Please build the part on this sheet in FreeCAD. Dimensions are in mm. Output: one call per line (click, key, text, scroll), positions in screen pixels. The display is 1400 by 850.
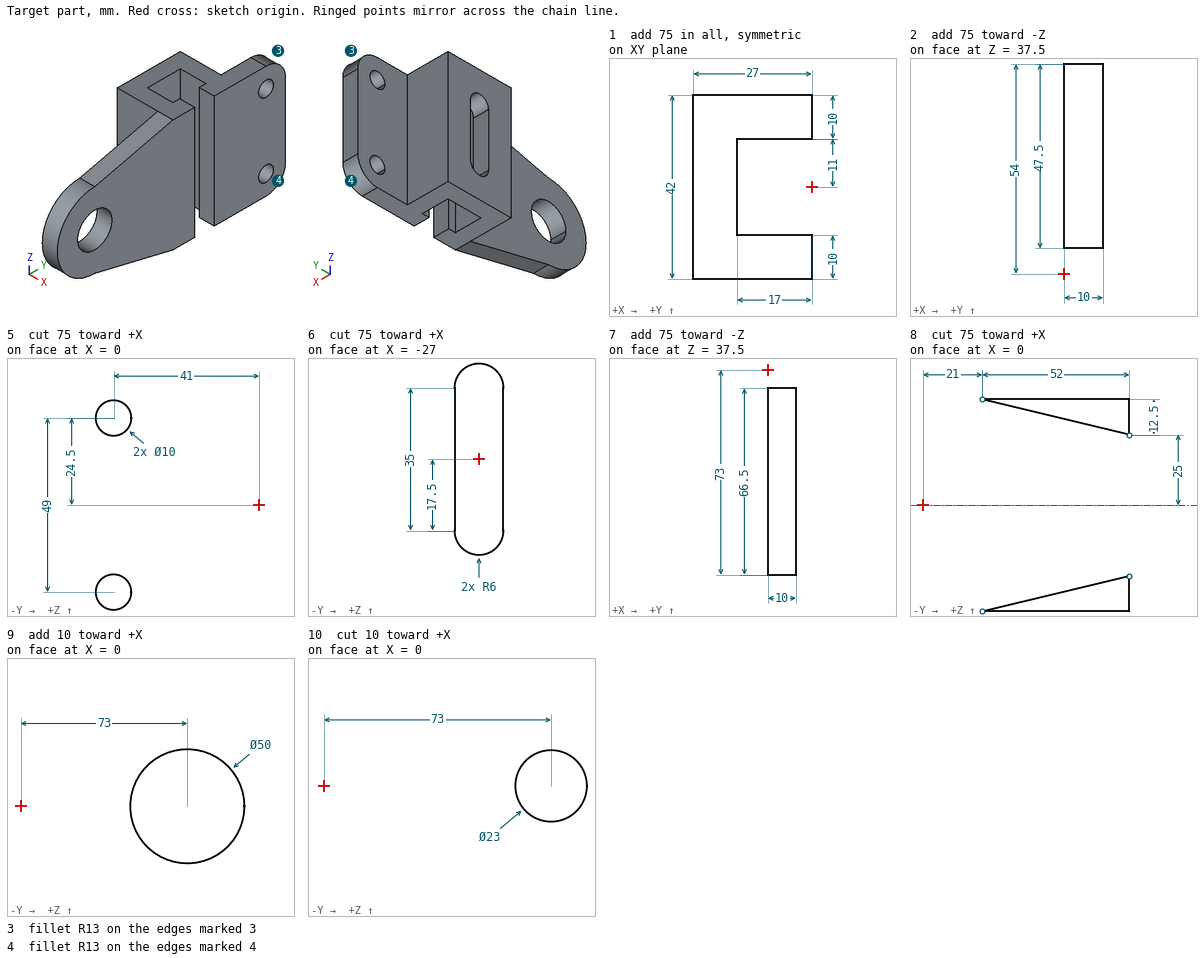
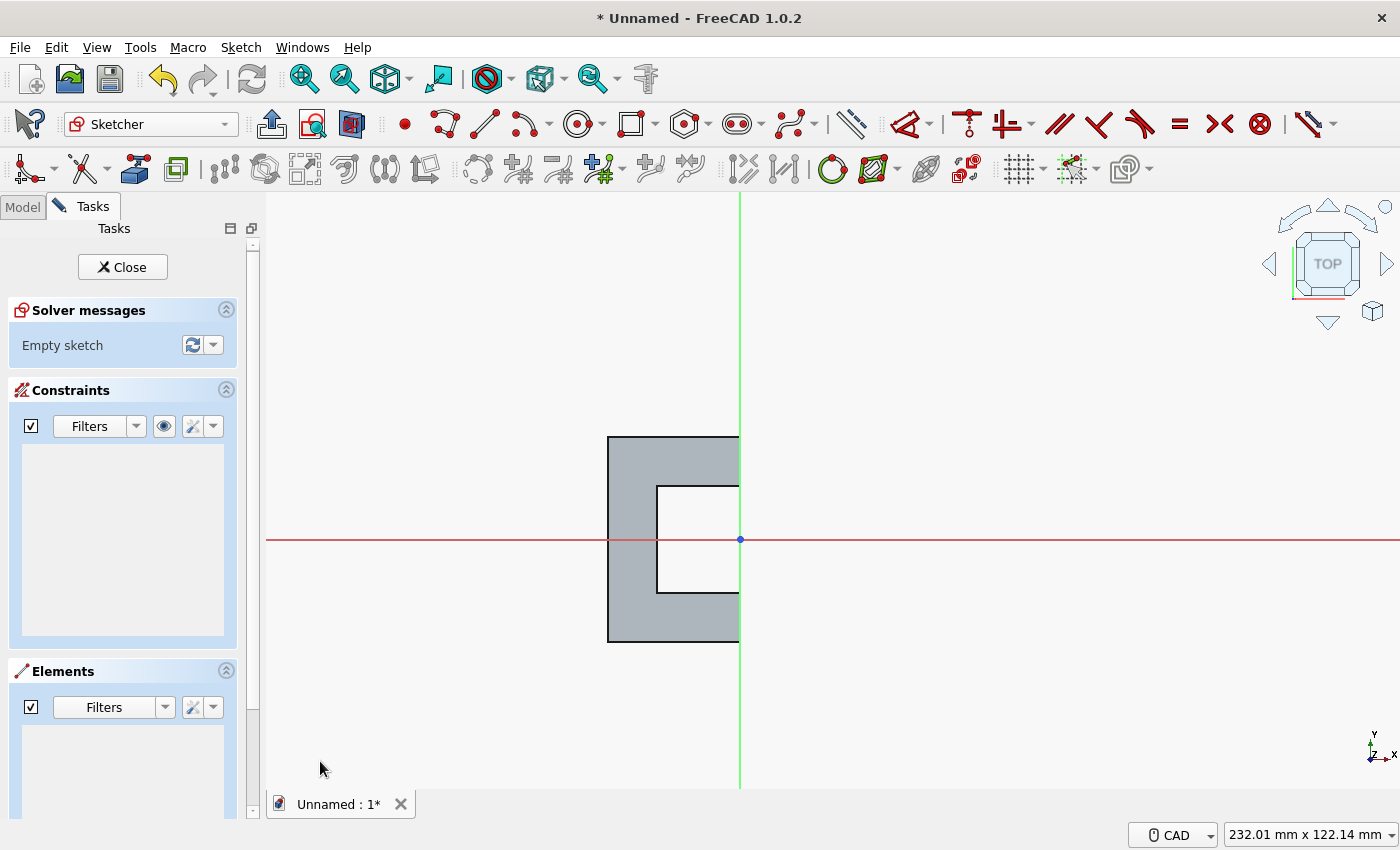
scroll(764, 239, up, 2)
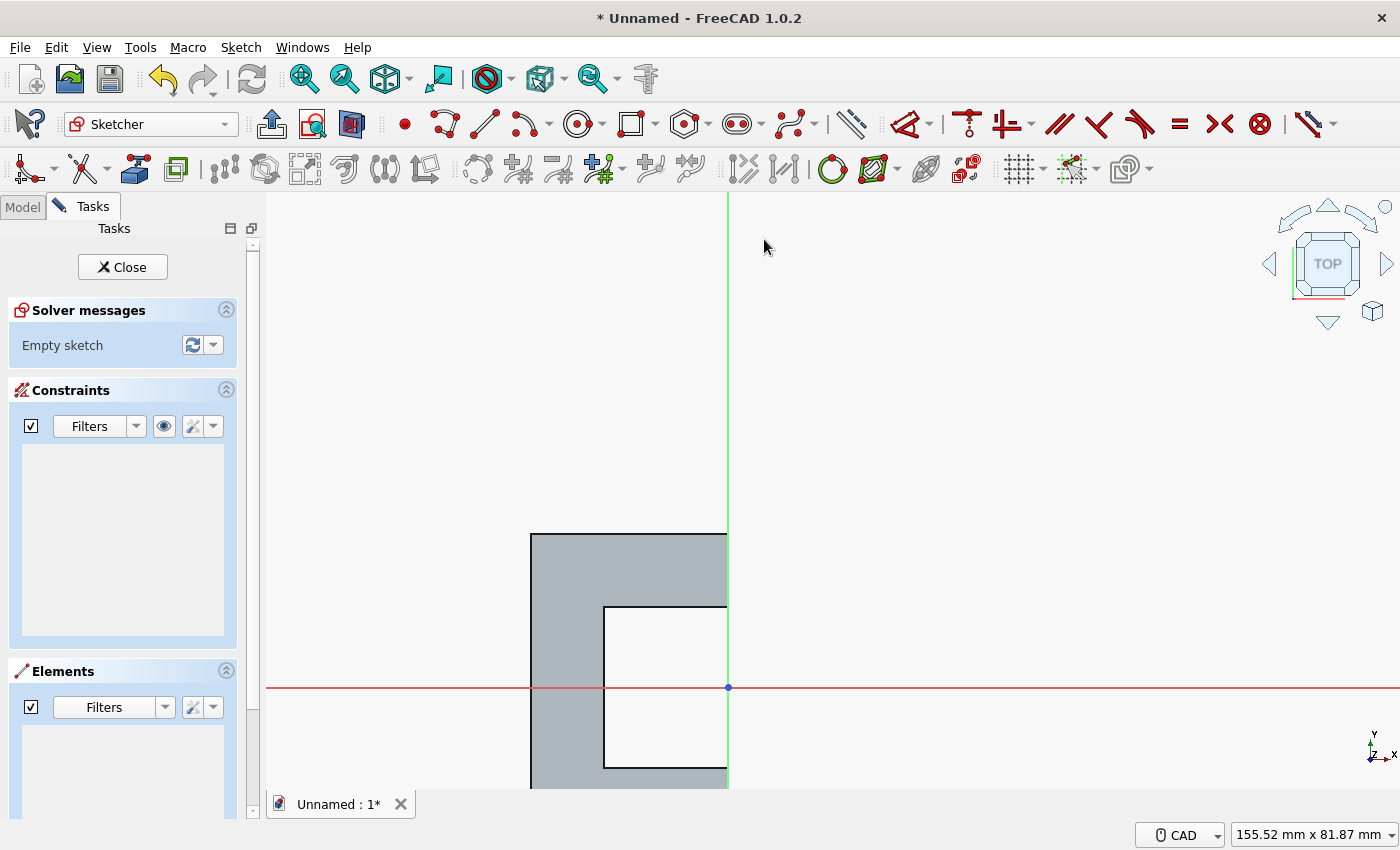
key(g)
key(r)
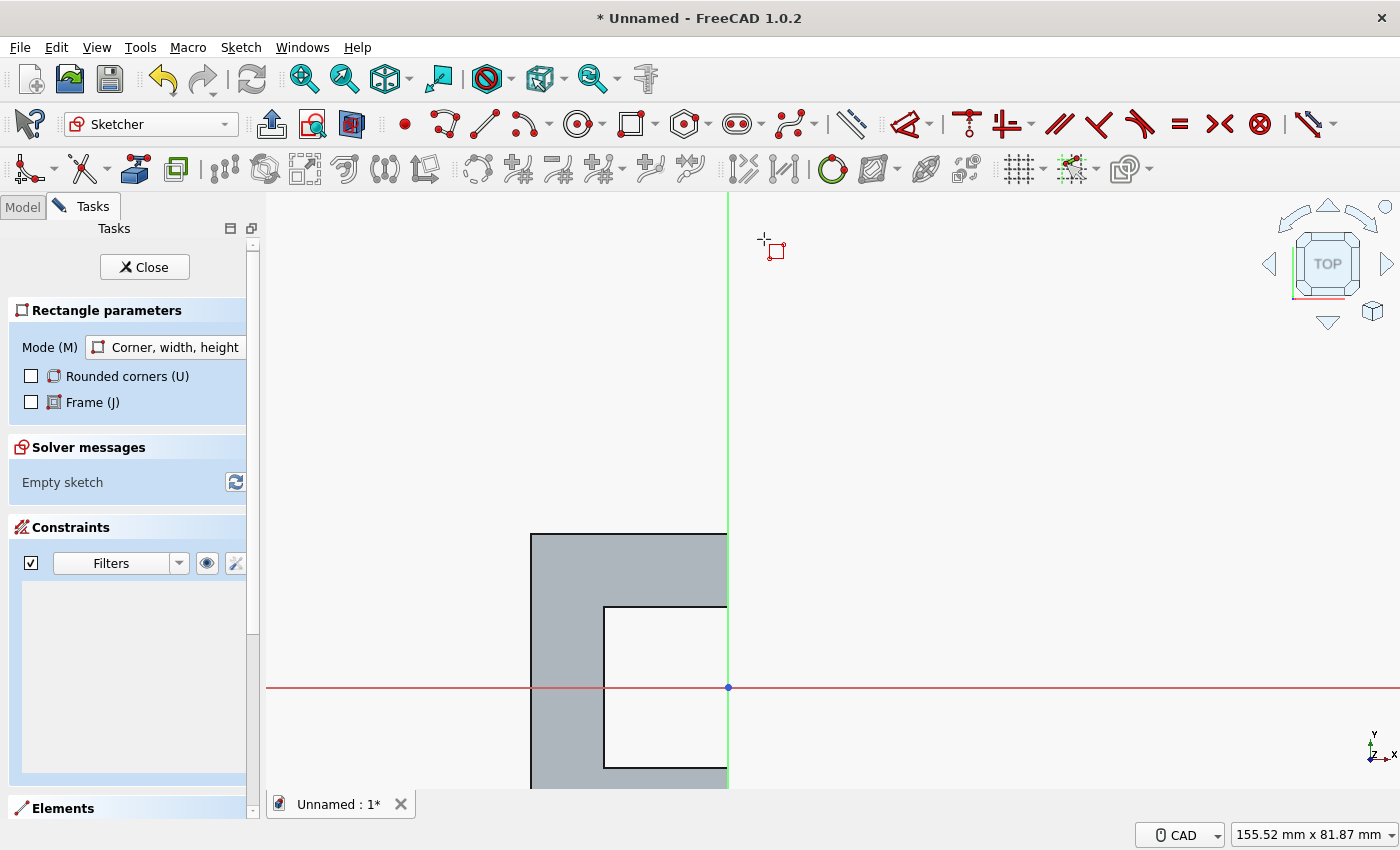
click(728, 294)
click(801, 640)
key(Escape)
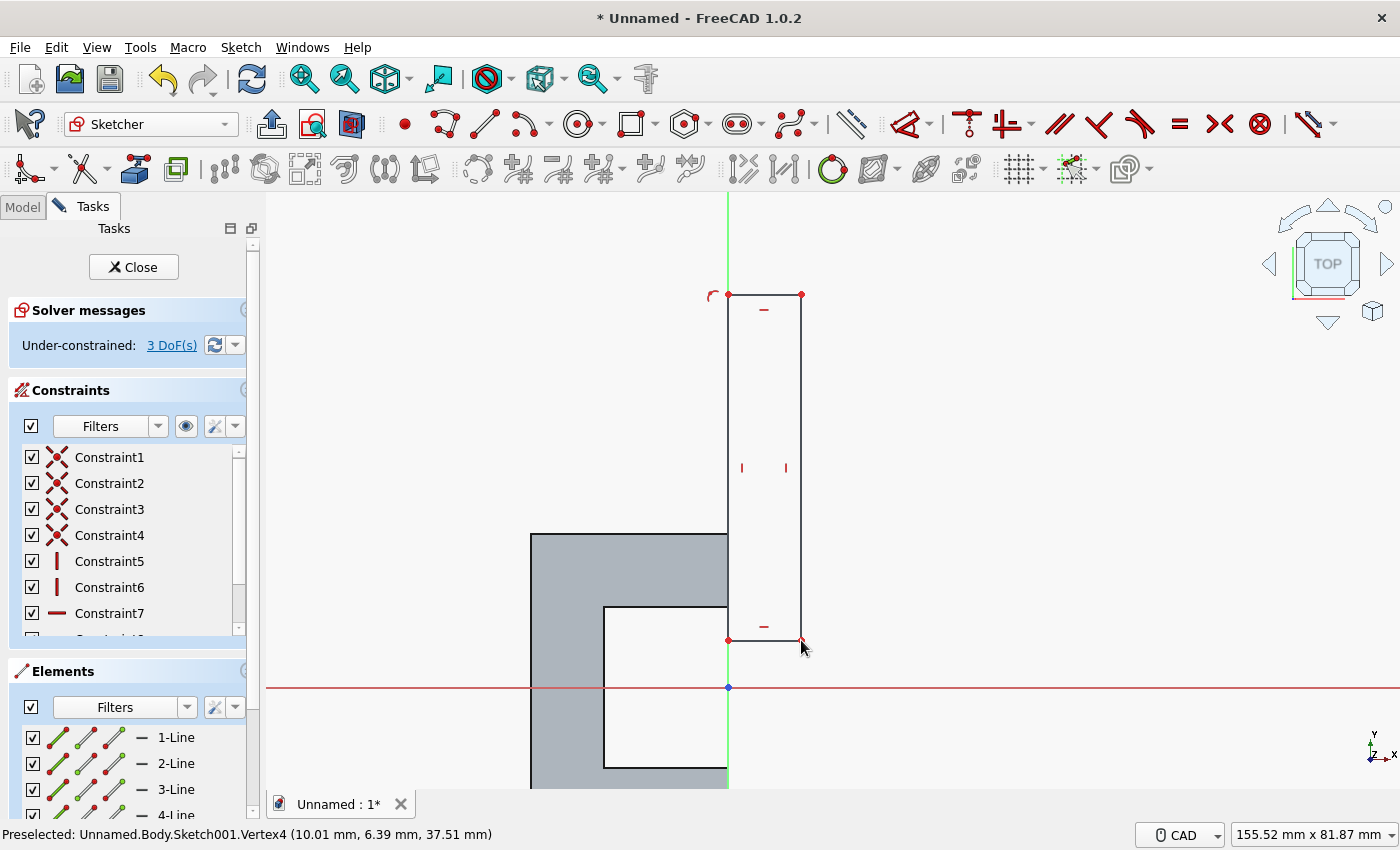
key(d)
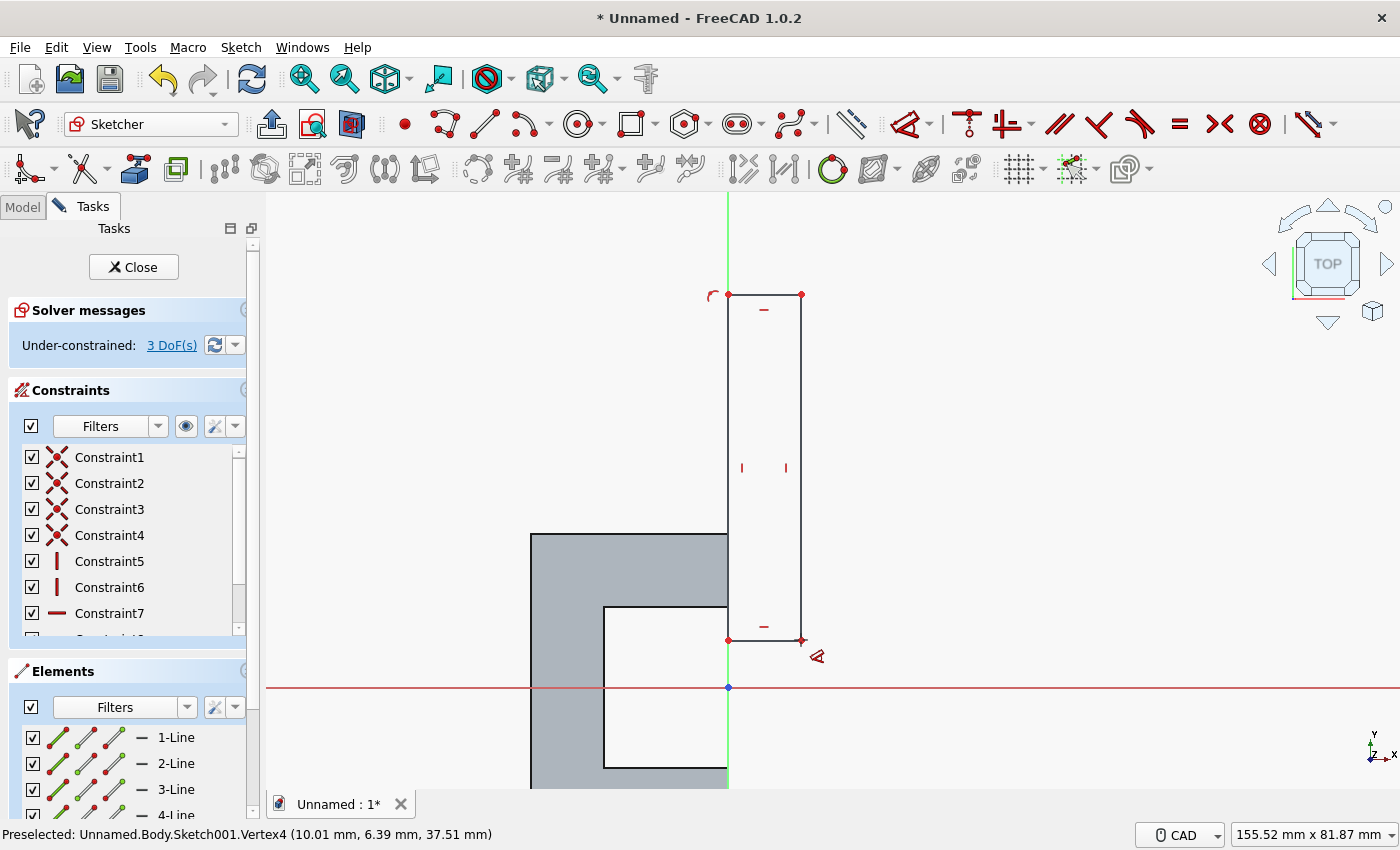
click(750, 641)
click(765, 607)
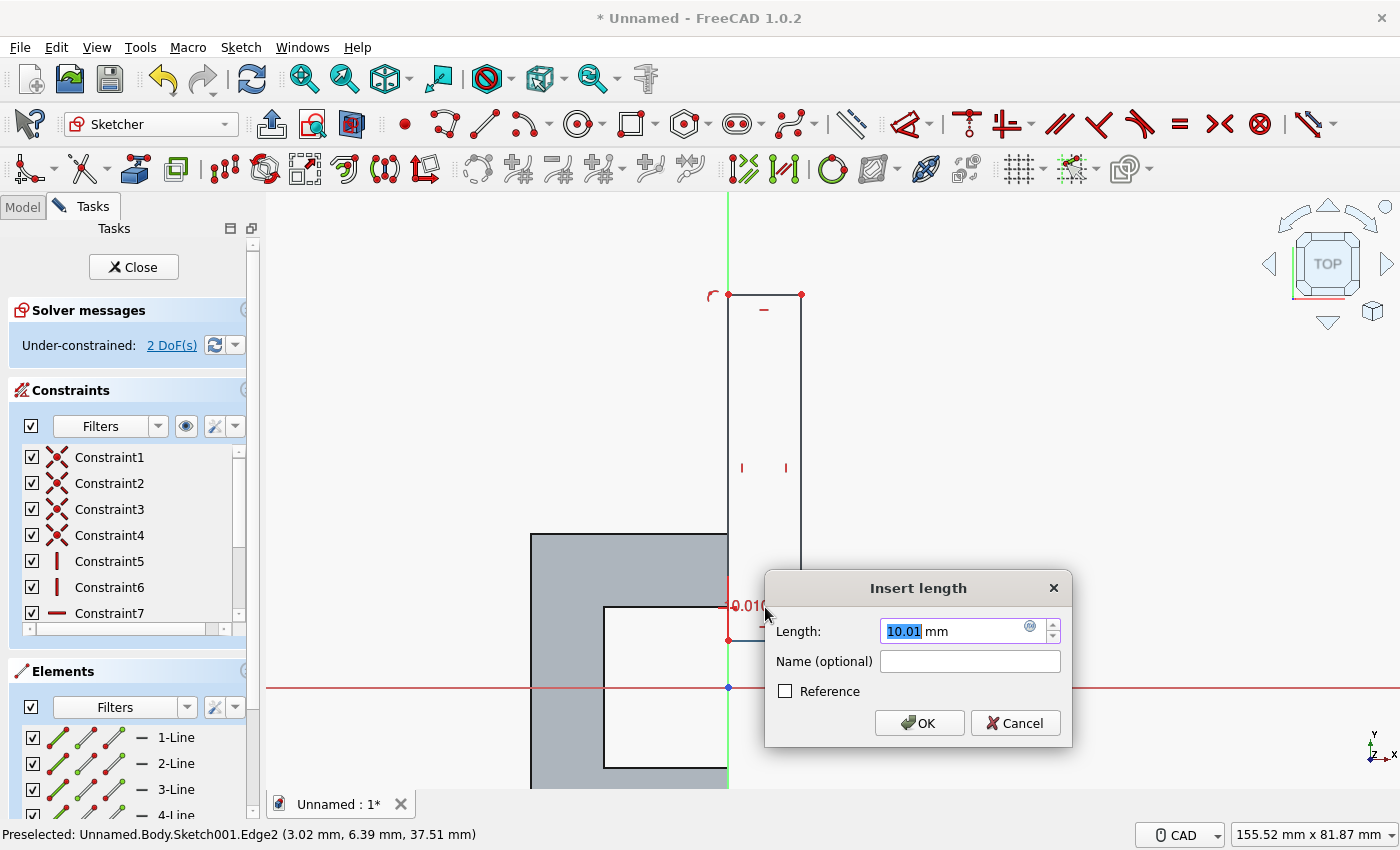
text(10)
key(Return)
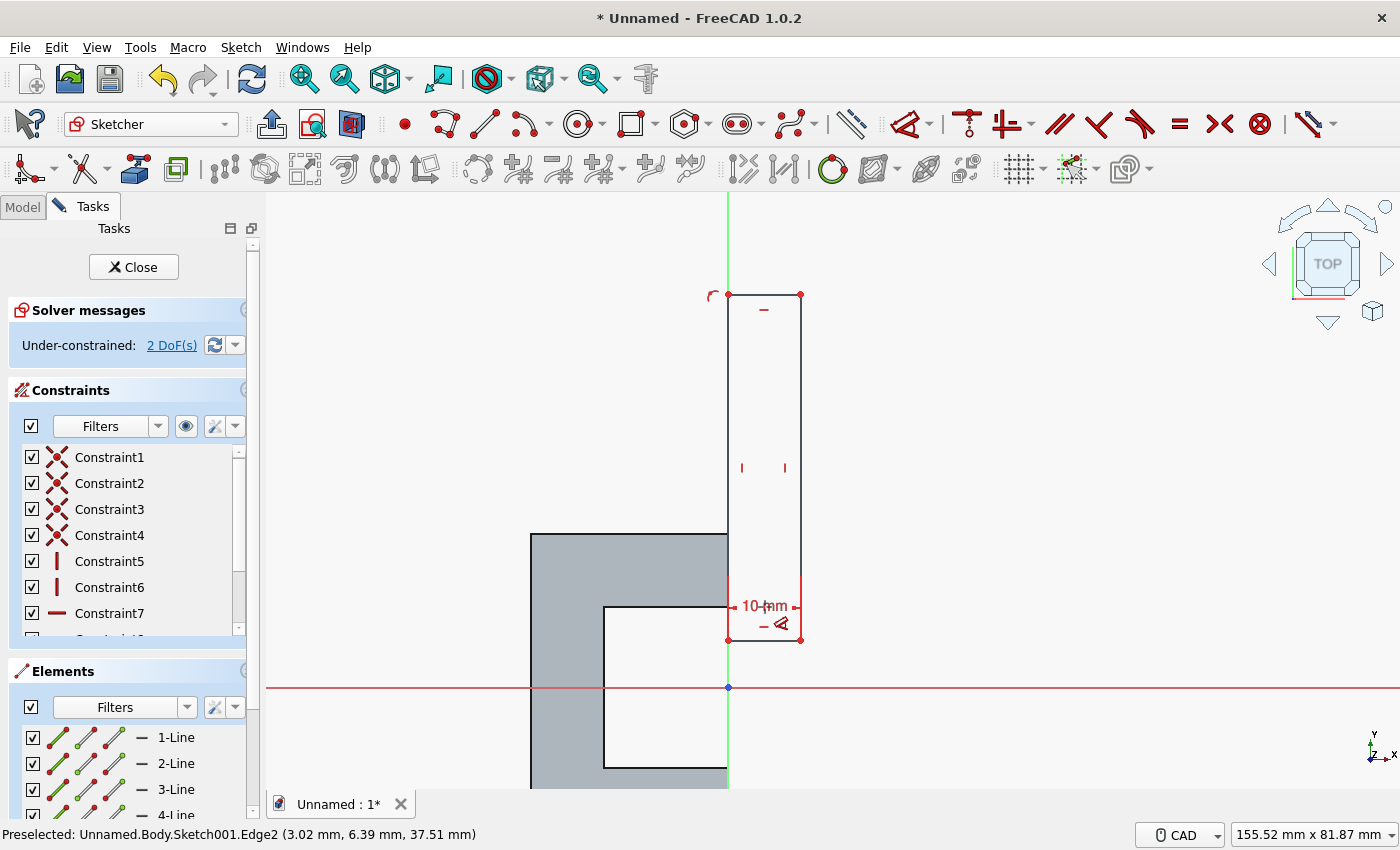
click(728, 295)
click(694, 491)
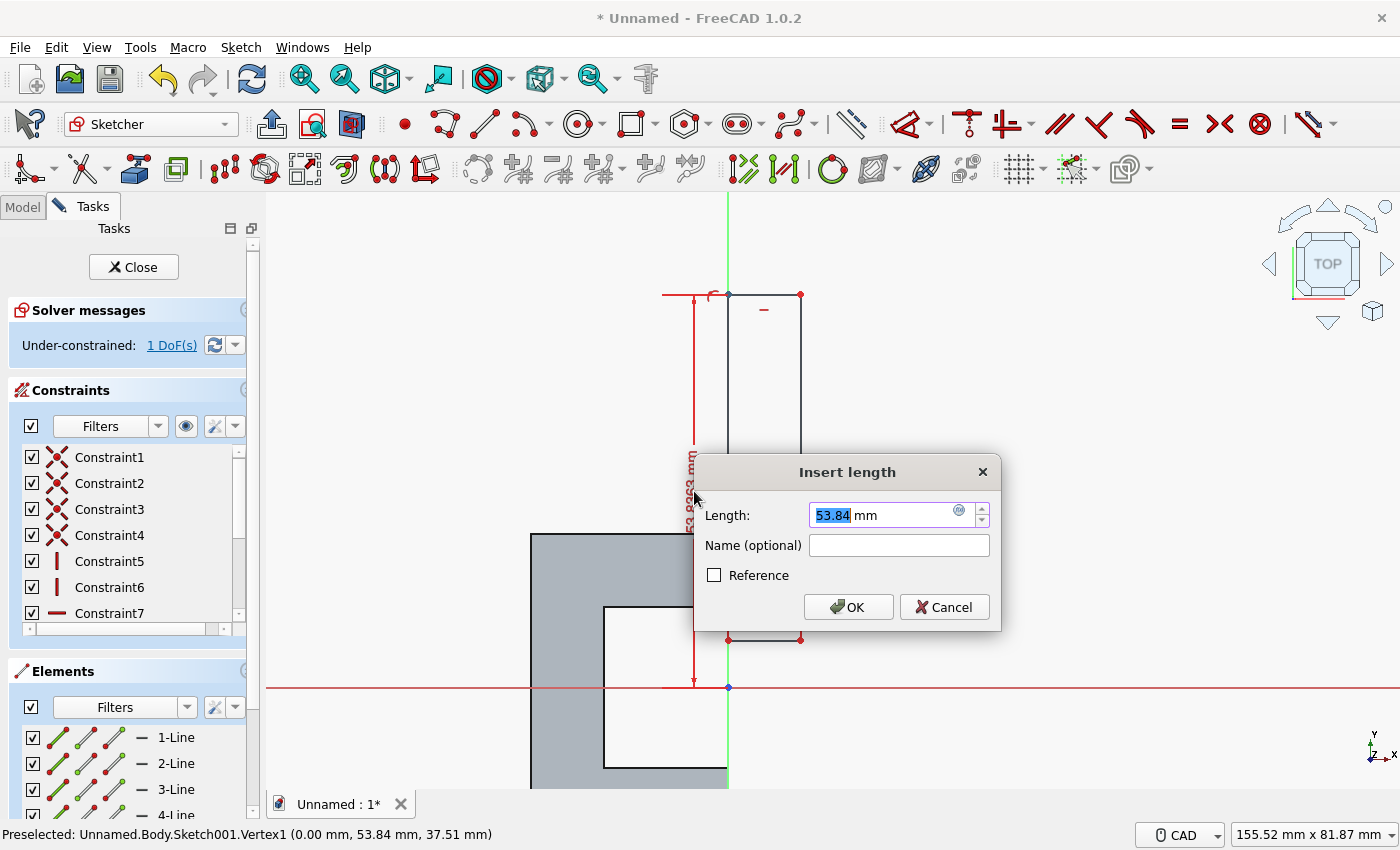
text(54)
key(Return)